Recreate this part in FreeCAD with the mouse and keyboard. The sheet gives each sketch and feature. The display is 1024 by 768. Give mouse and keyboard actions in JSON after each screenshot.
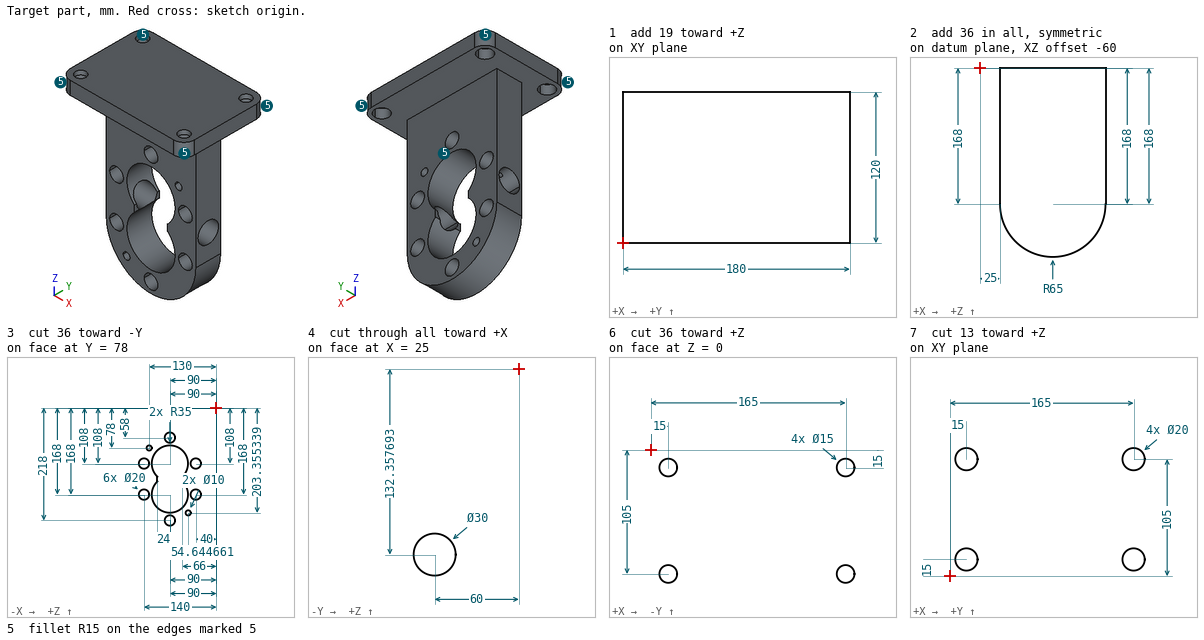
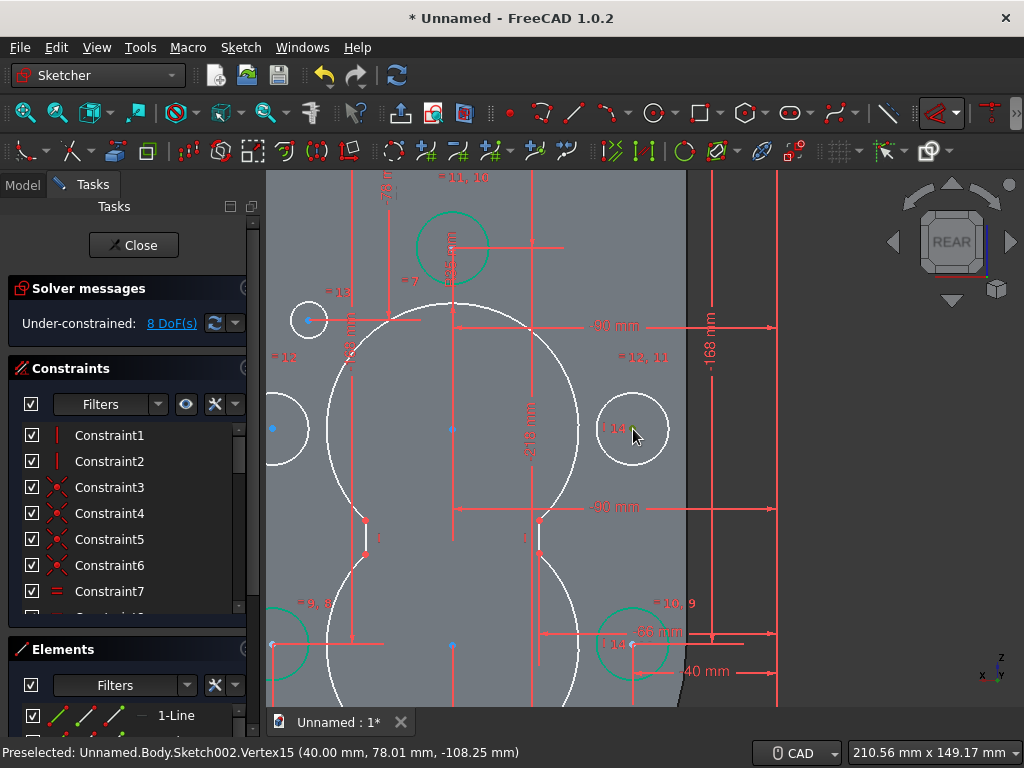
{"action": "key", "text": "i"}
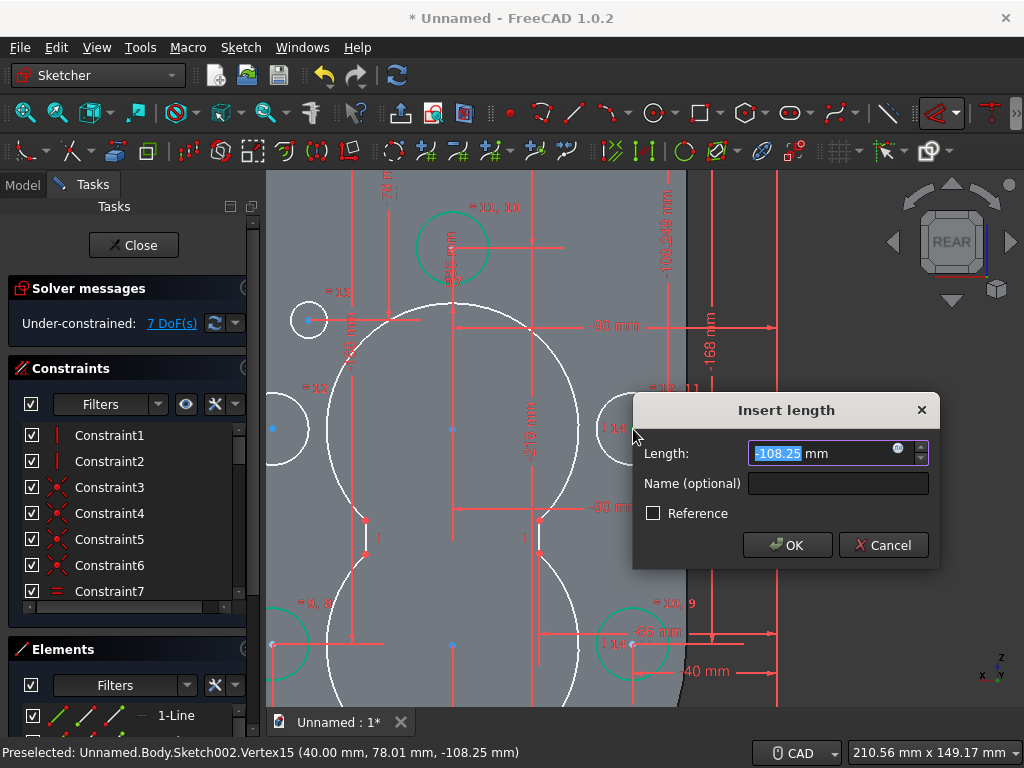
{"action": "type", "text": "-108"}
{"action": "key", "text": "Return"}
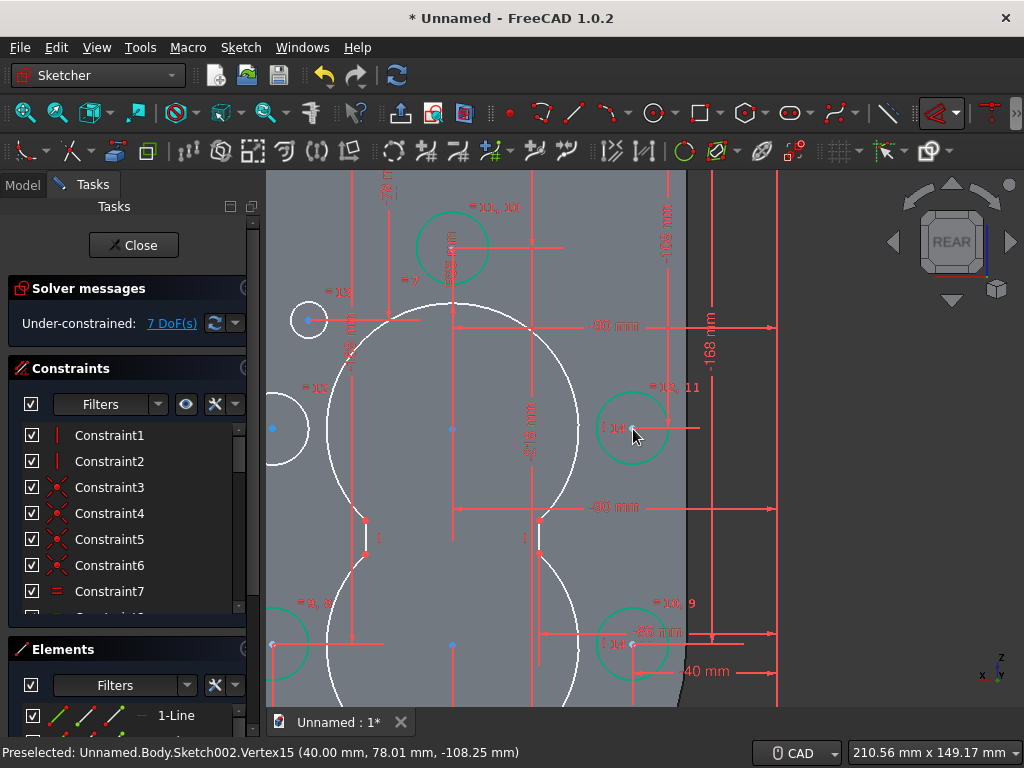
{"action": "scroll", "coordinate": [634, 429], "scroll_direction": "down", "scroll_amount": 4}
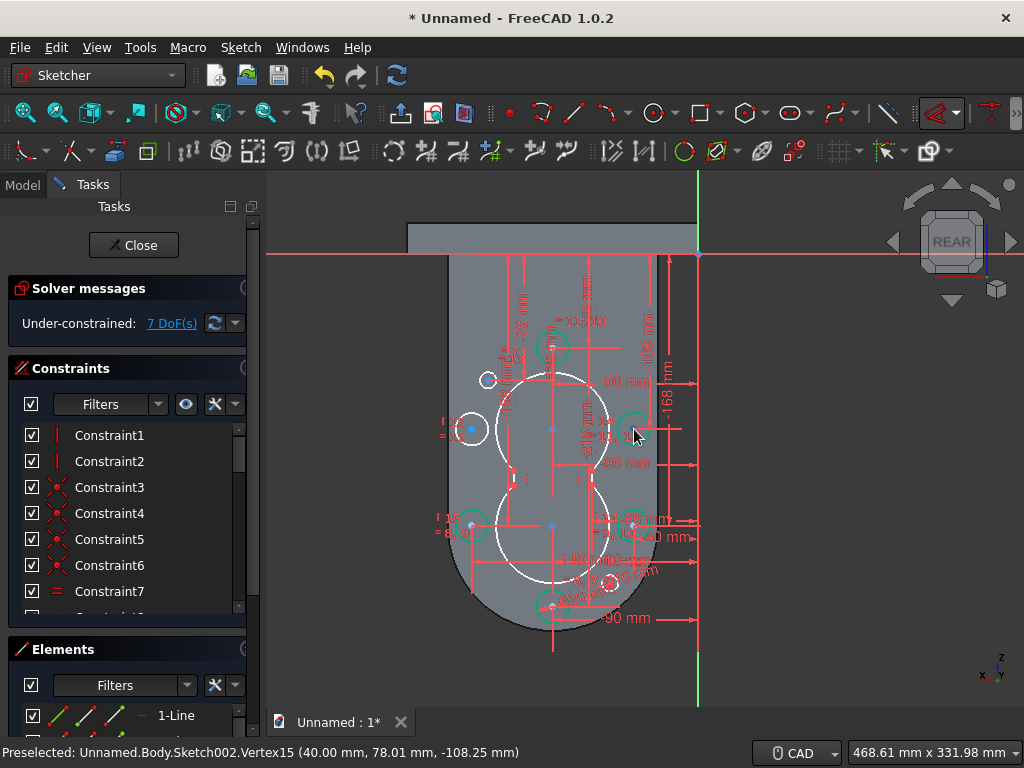
{"action": "left_click", "coordinate": [472, 429]}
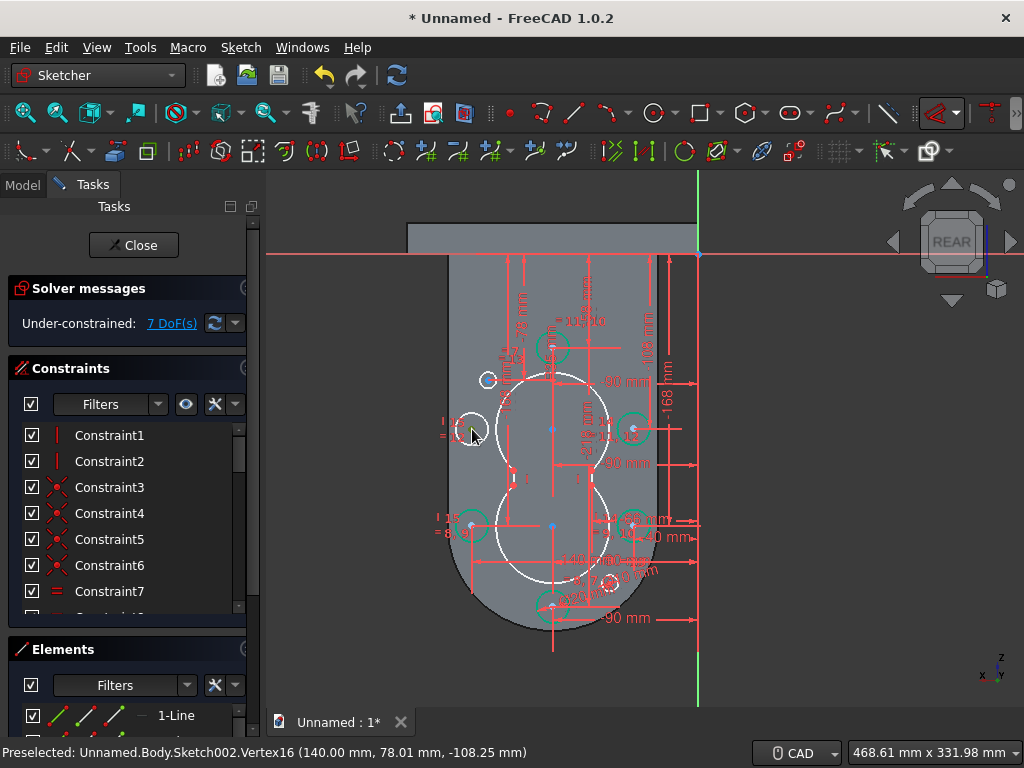
{"action": "left_click", "coordinate": [958, 114]}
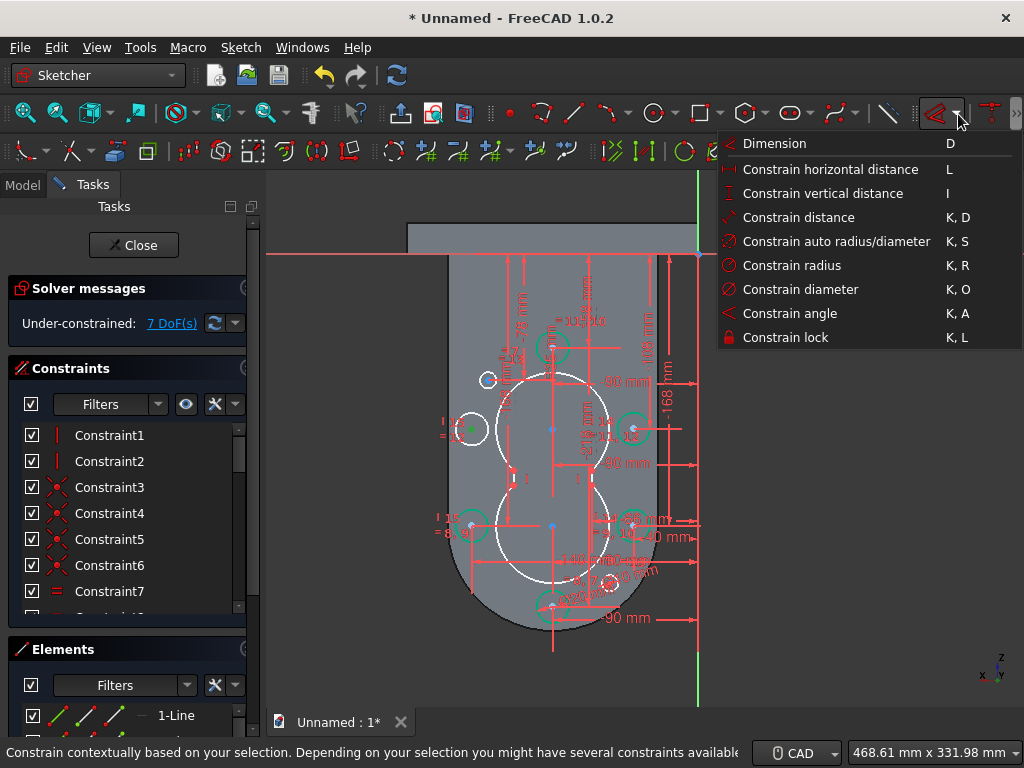
{"action": "left_click", "coordinate": [870, 193]}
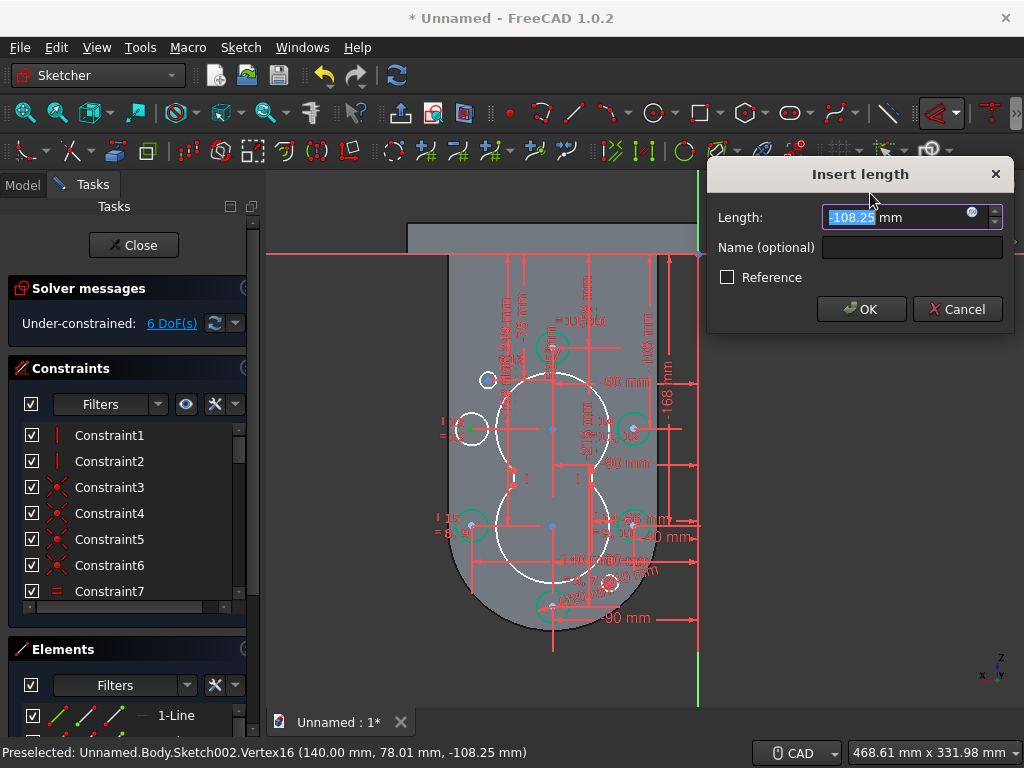
{"action": "type", "text": "-108"}
{"action": "key", "text": "Return"}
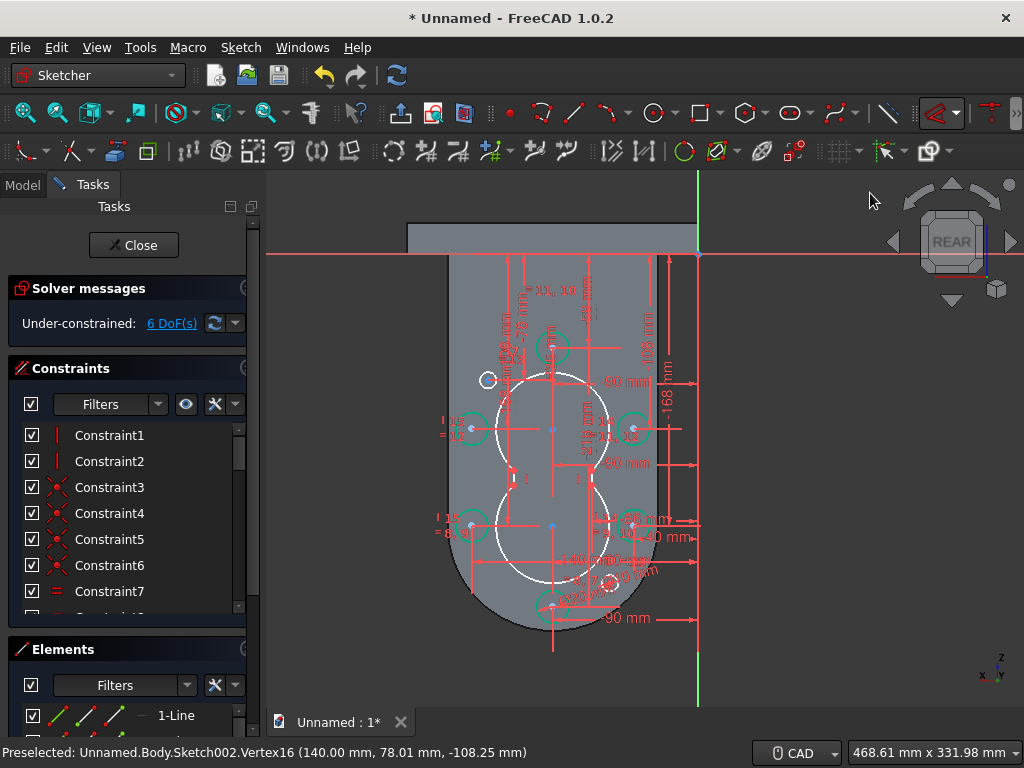
{"action": "left_click", "coordinate": [488, 380]}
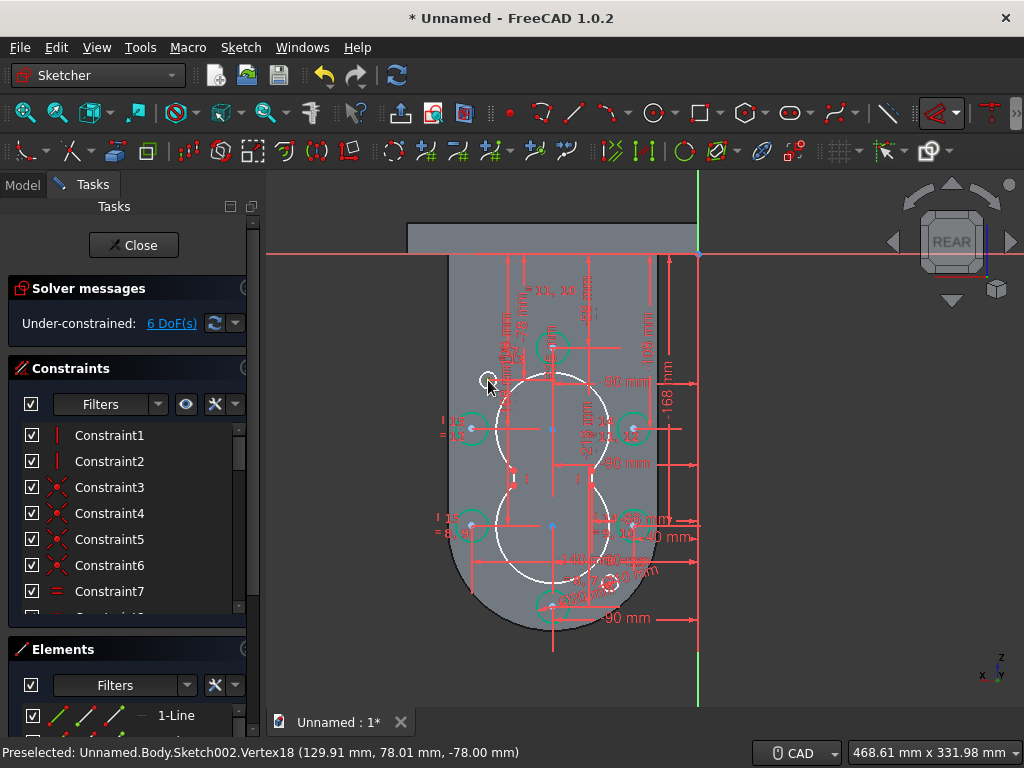
{"action": "key", "text": "l"}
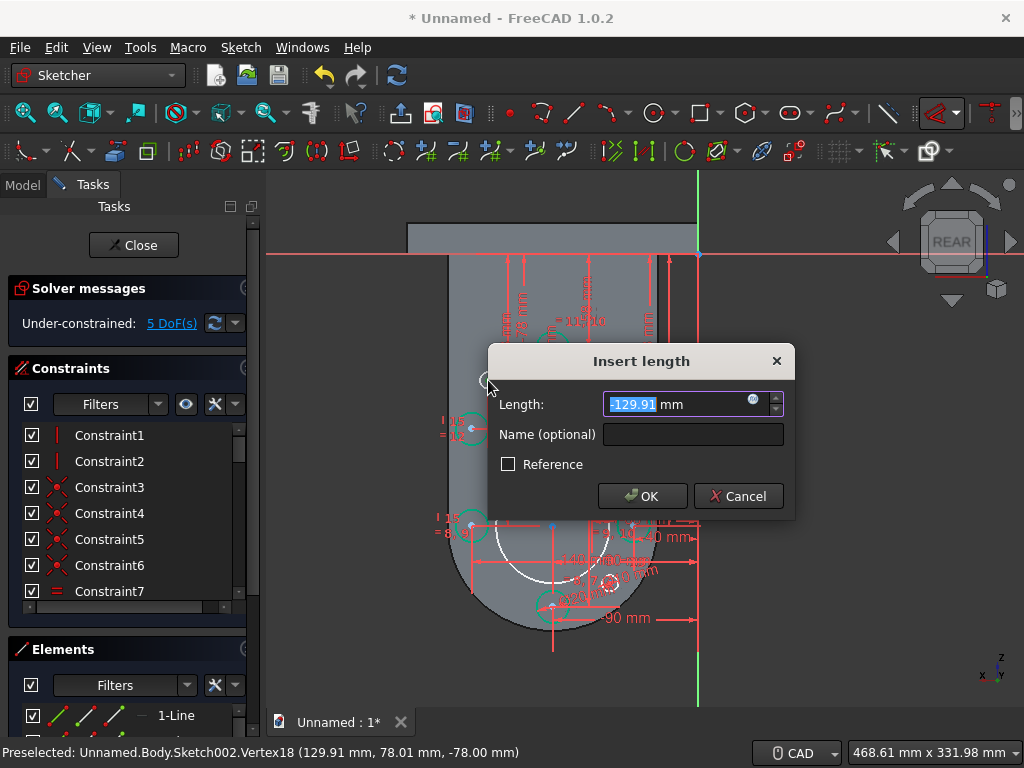
{"action": "type", "text": "-130"}
{"action": "key", "text": "Return"}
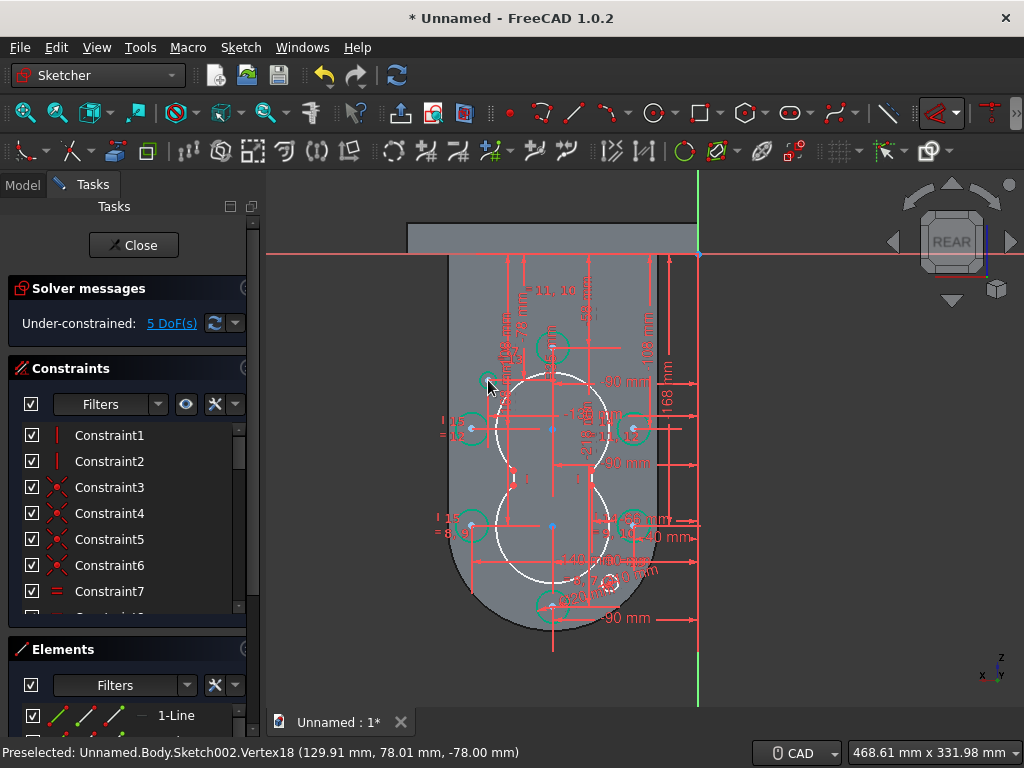
{"action": "left_click", "coordinate": [514, 486]}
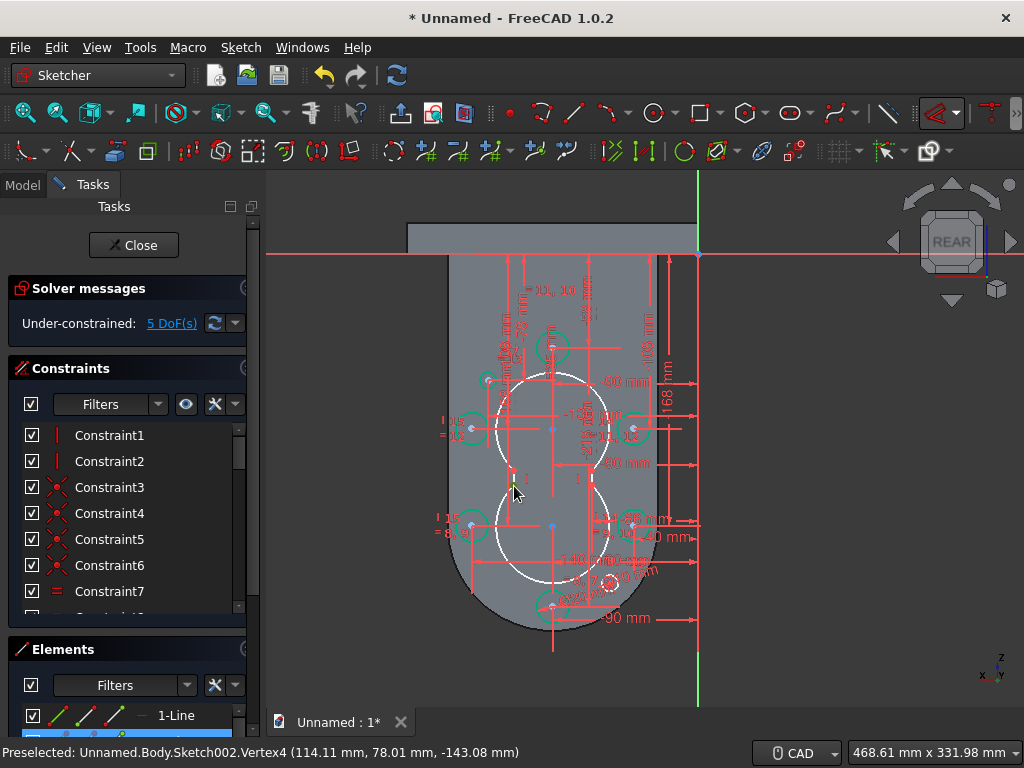
{"action": "left_click", "coordinate": [553, 607]}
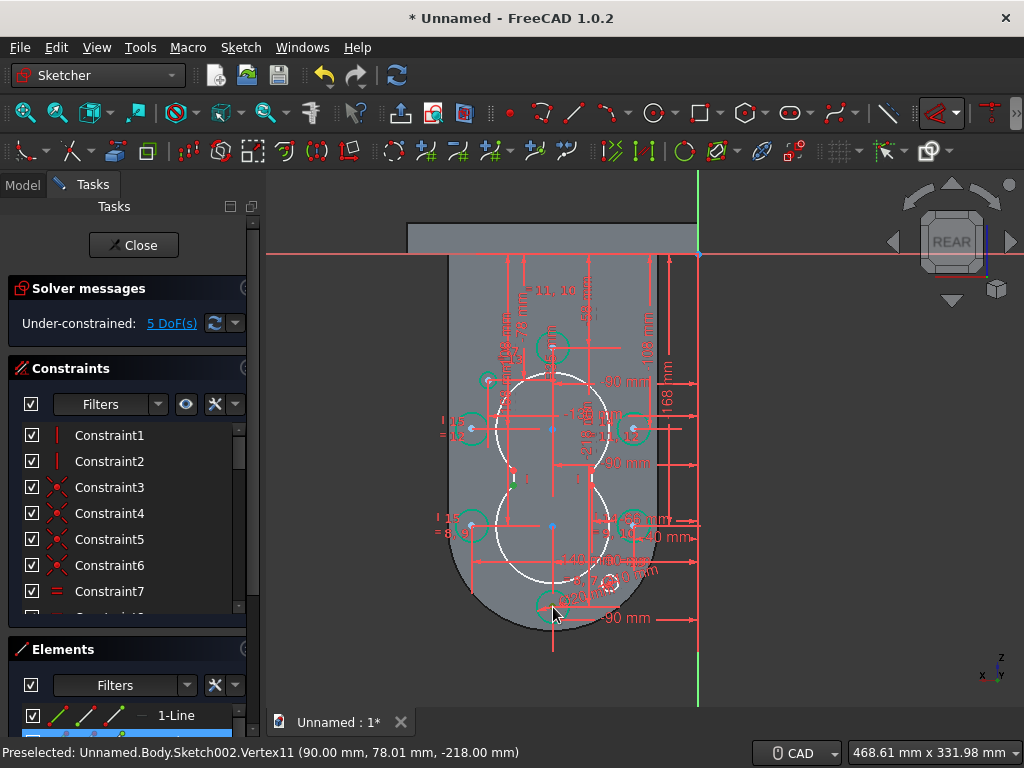
{"action": "left_click", "coordinate": [958, 114]}